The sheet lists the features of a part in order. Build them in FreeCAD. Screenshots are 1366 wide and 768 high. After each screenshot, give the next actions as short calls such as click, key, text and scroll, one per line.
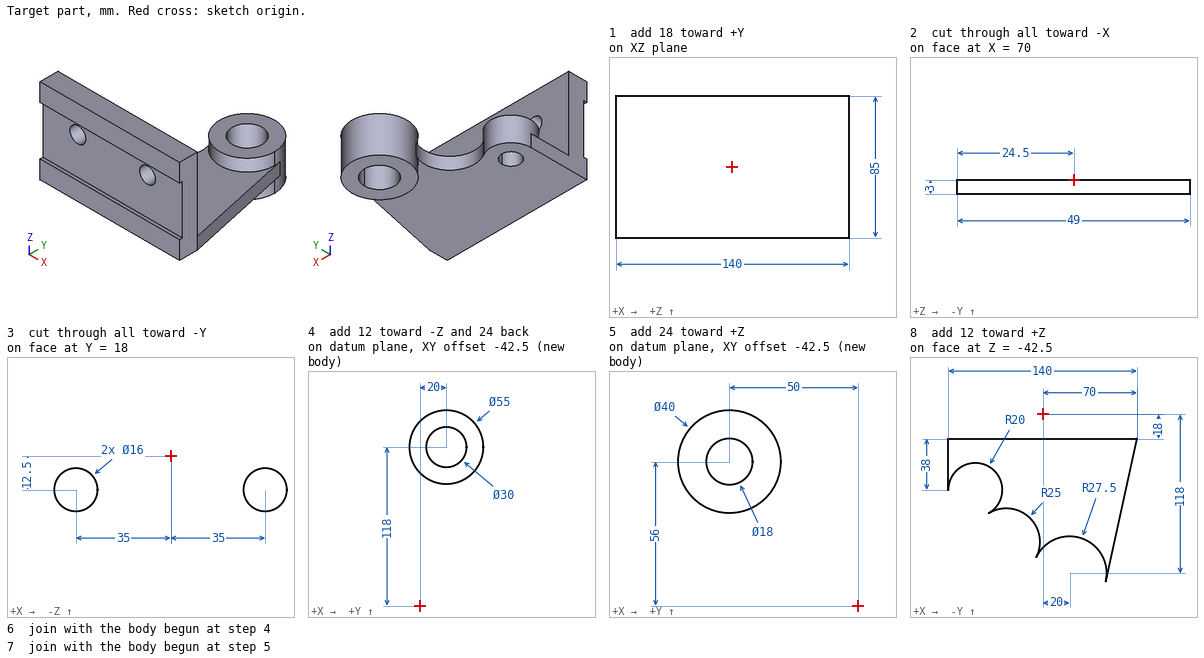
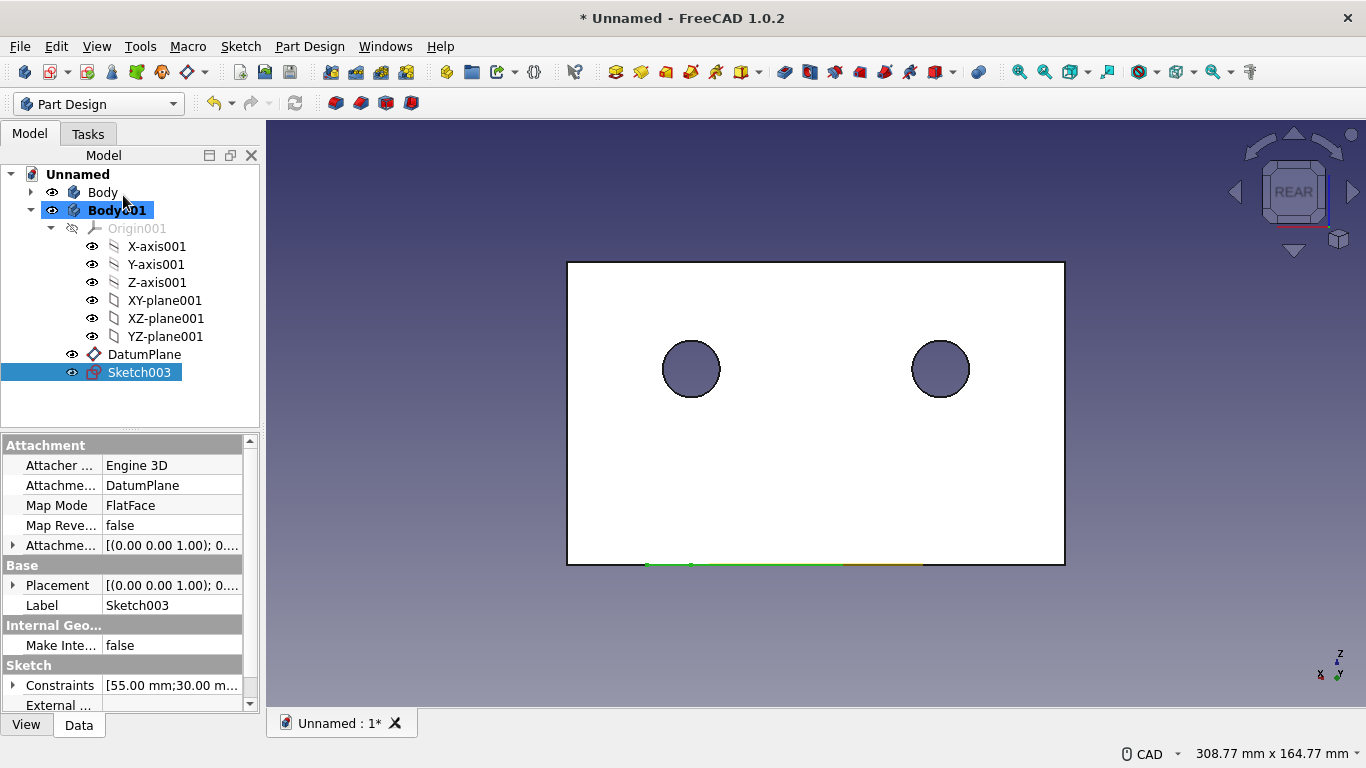
click(616, 72)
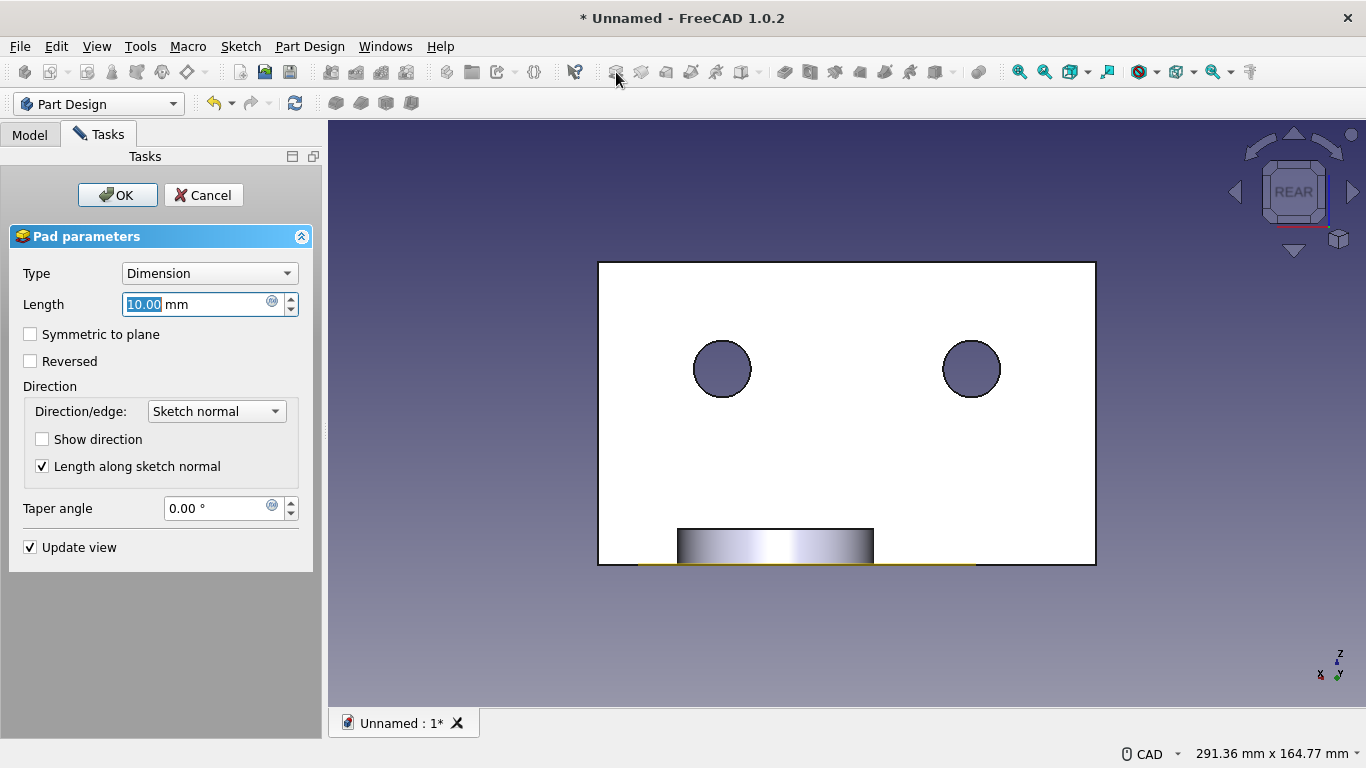
click(210, 274)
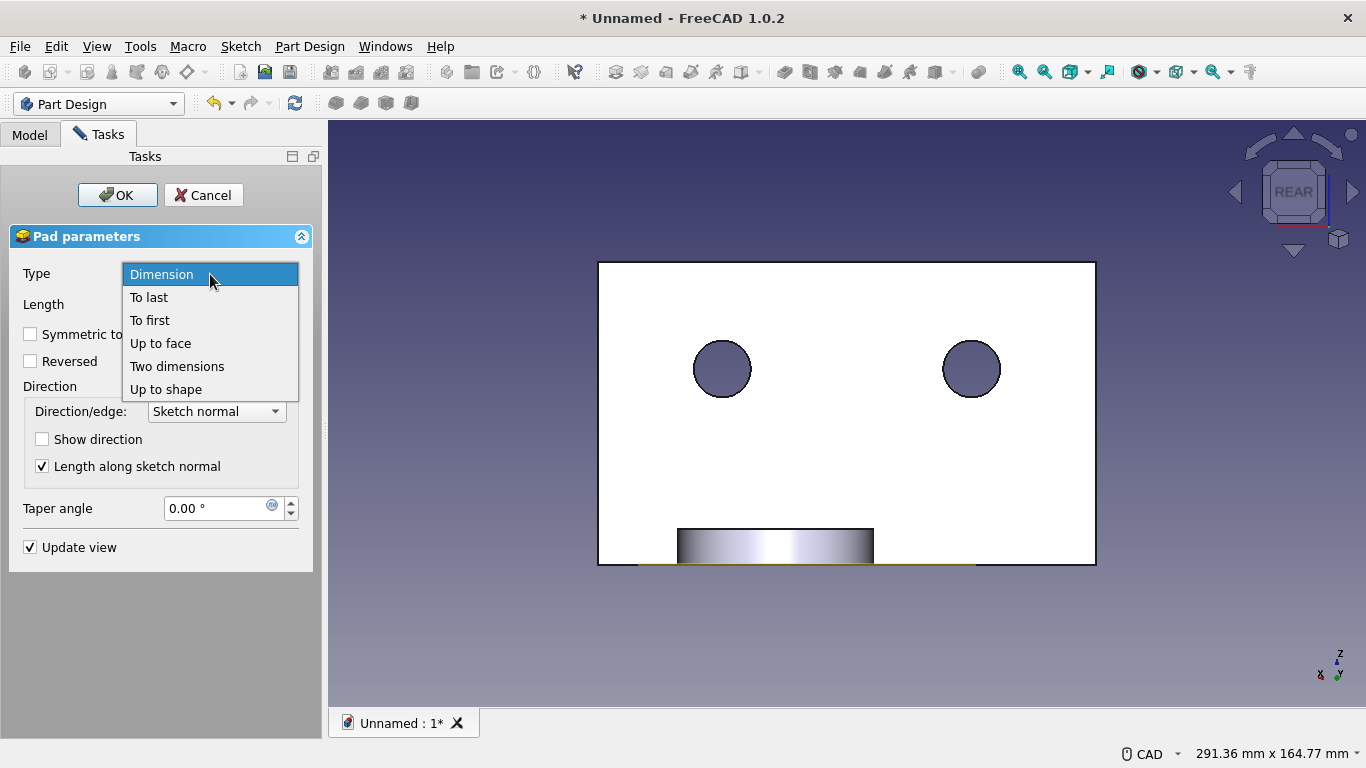
click(208, 366)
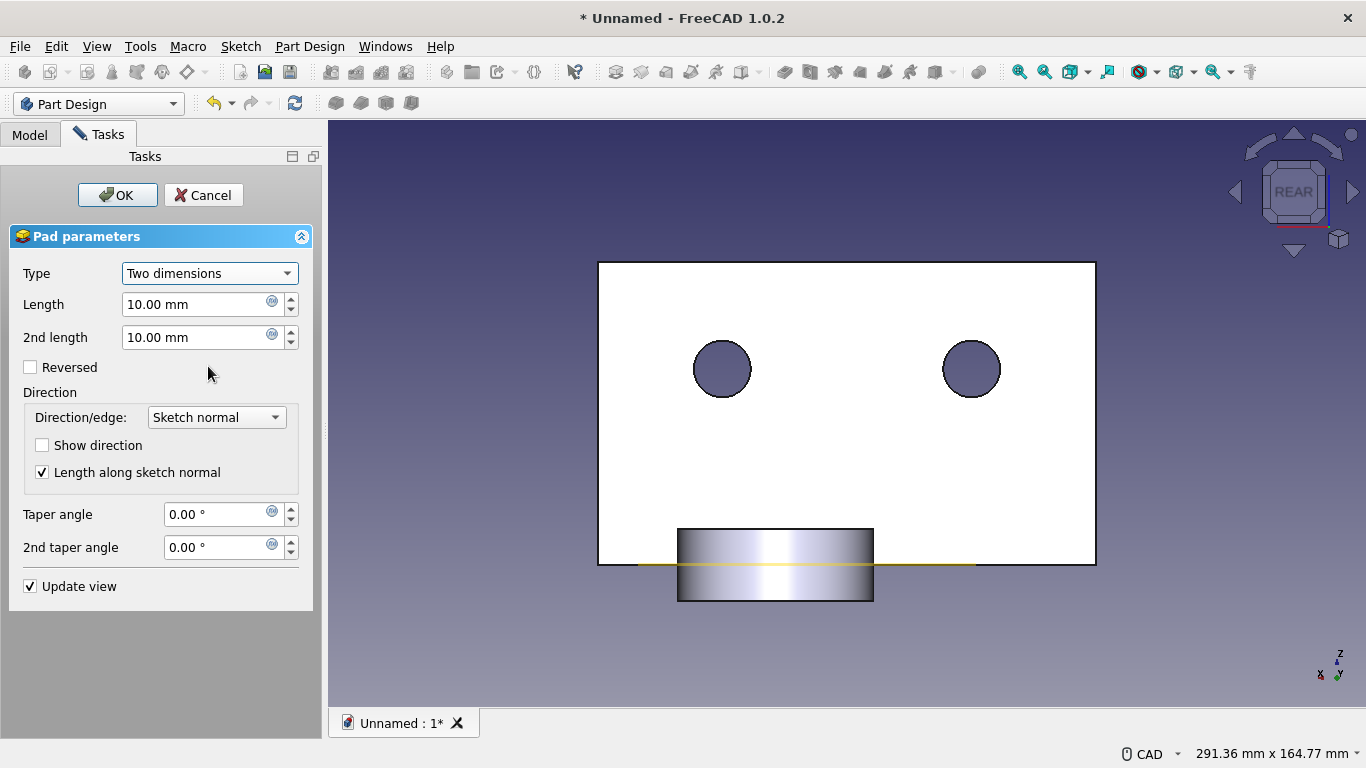
triple_click(204, 304)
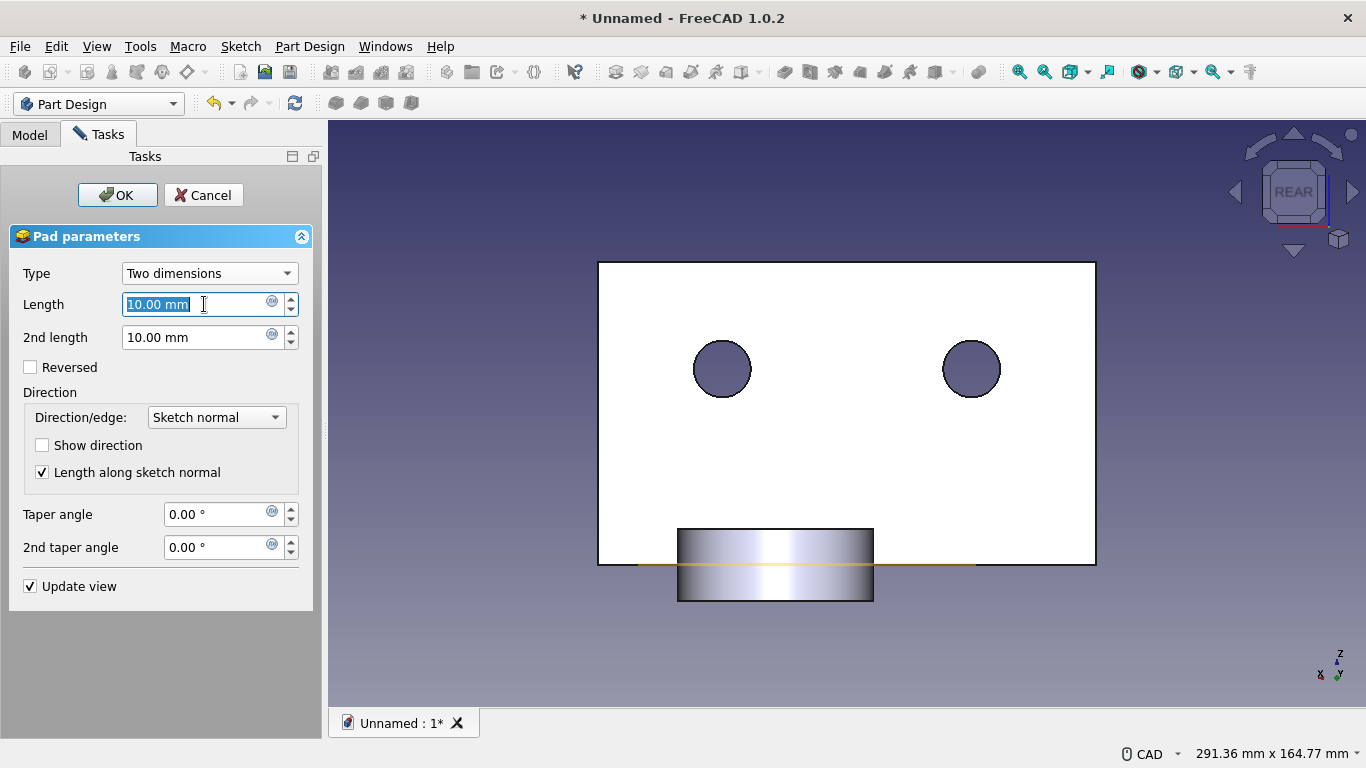
text(12)
key(Tab)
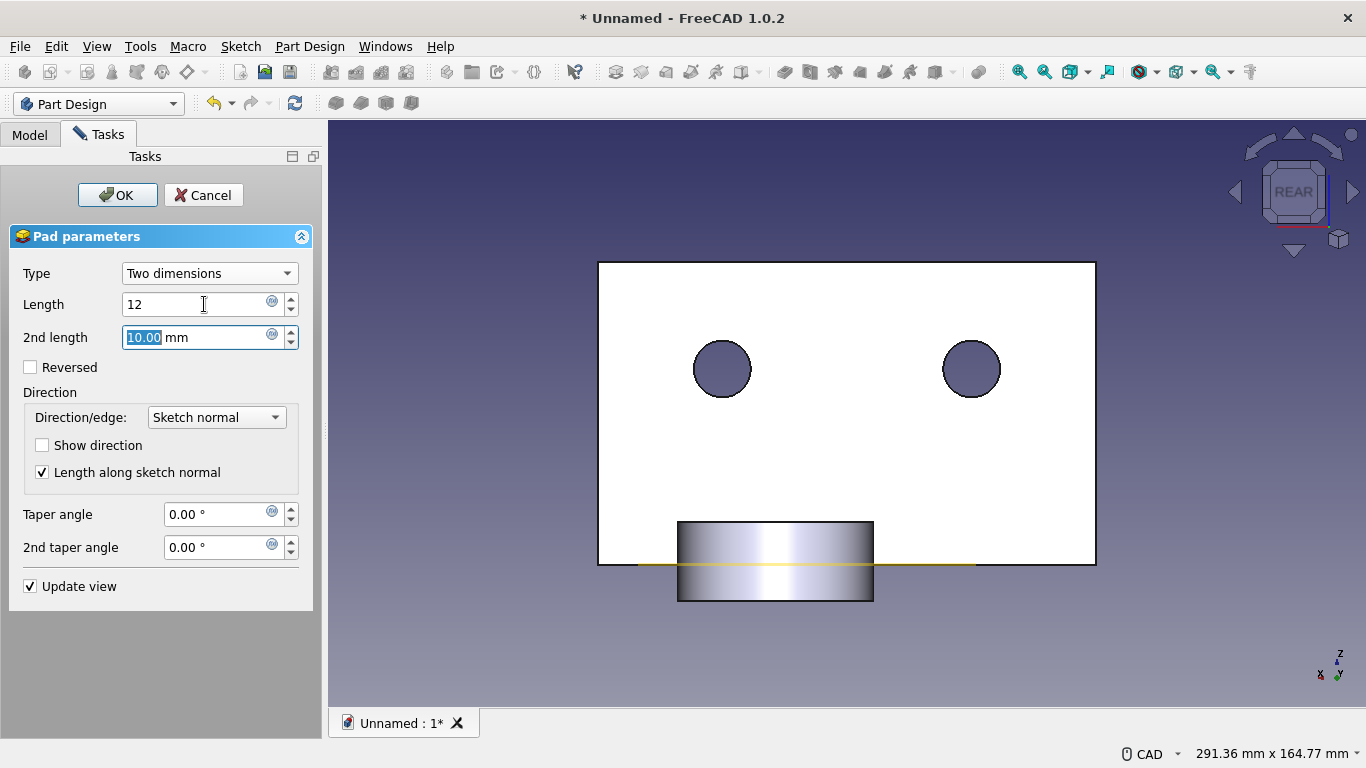
text(24)
key(Tab)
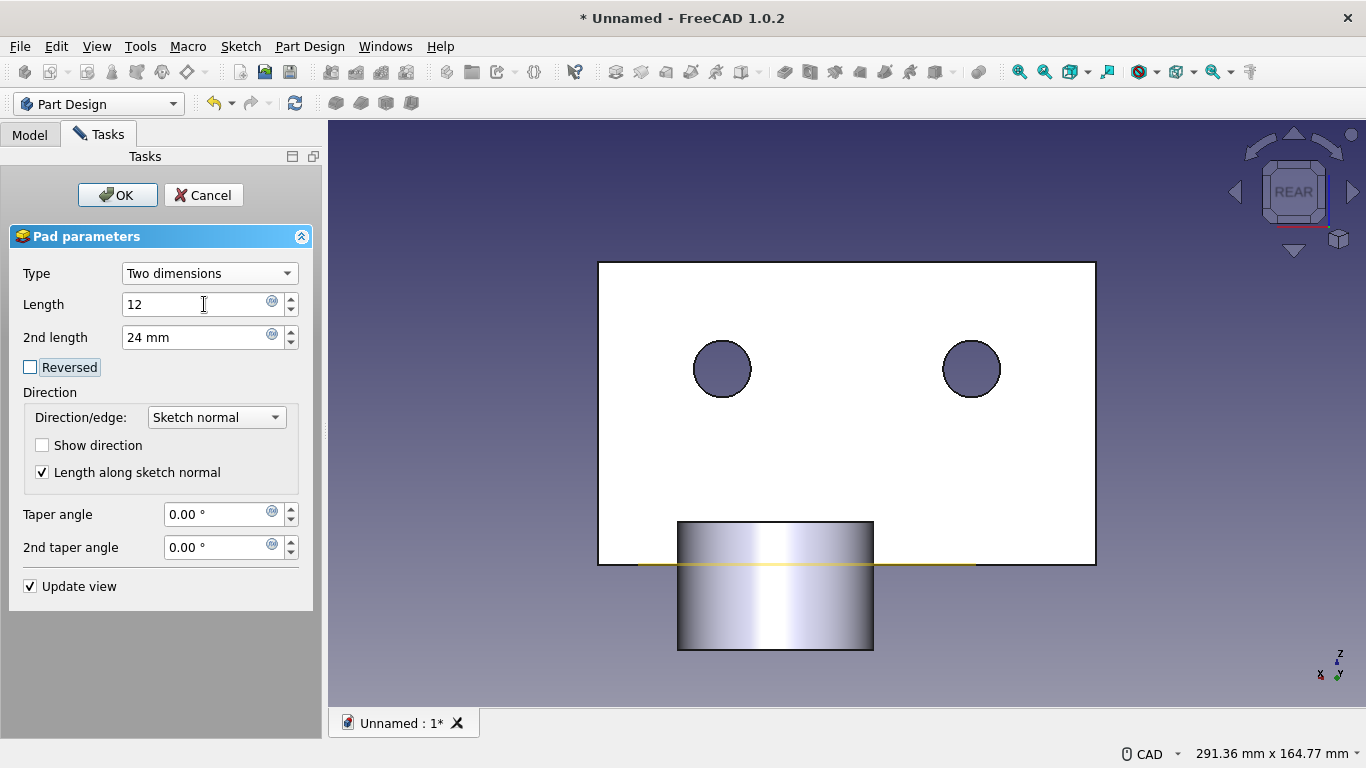
click(31, 367)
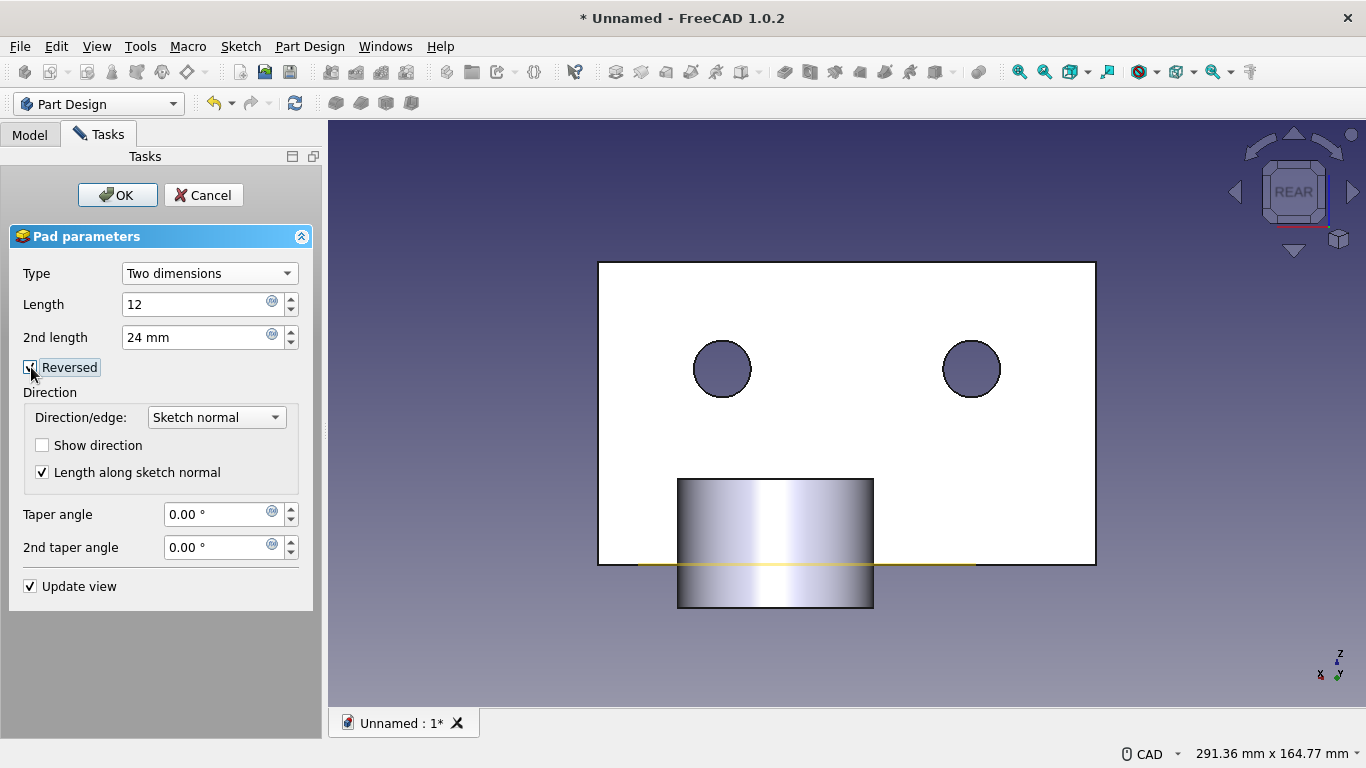
click(118, 195)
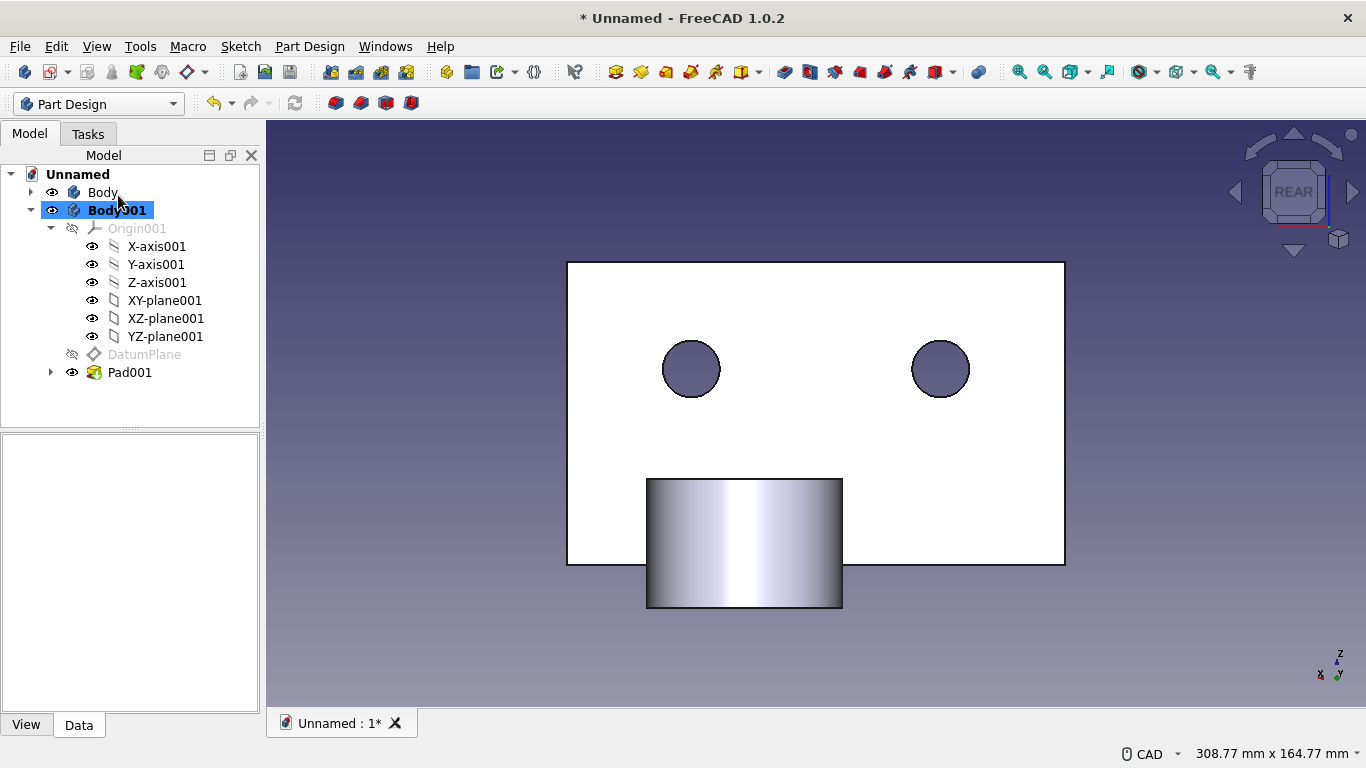
click(1020, 72)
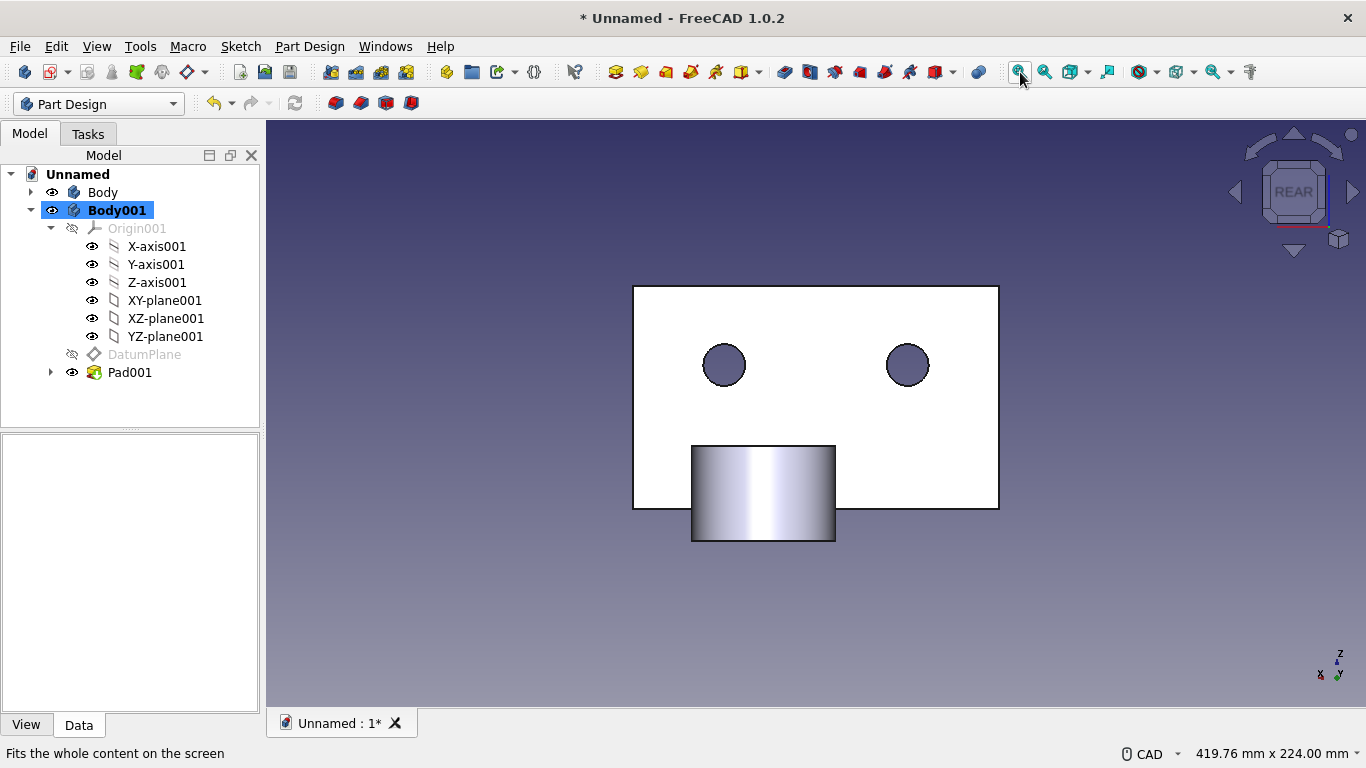
click(25, 72)